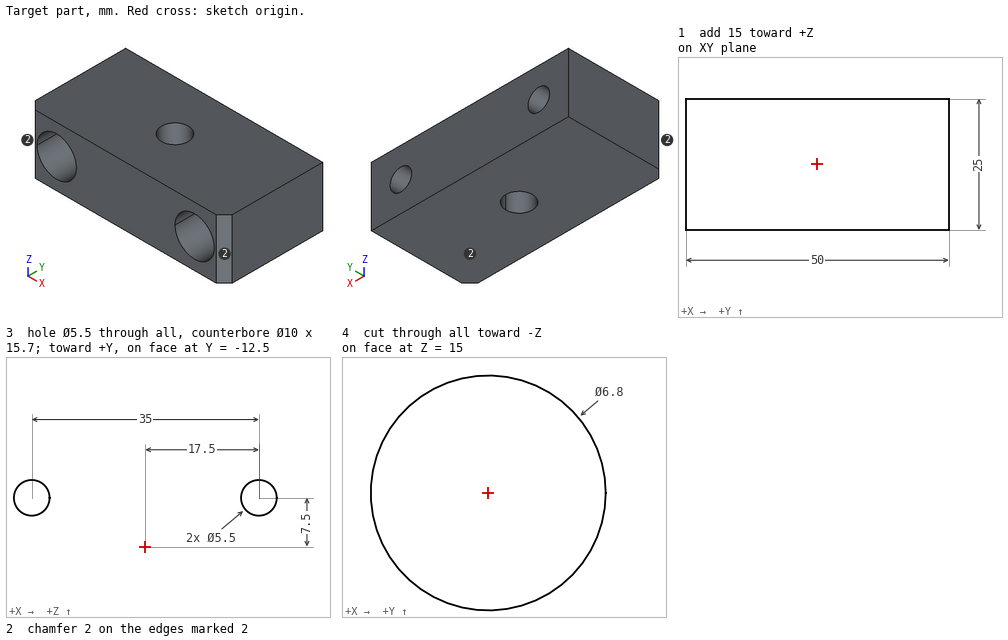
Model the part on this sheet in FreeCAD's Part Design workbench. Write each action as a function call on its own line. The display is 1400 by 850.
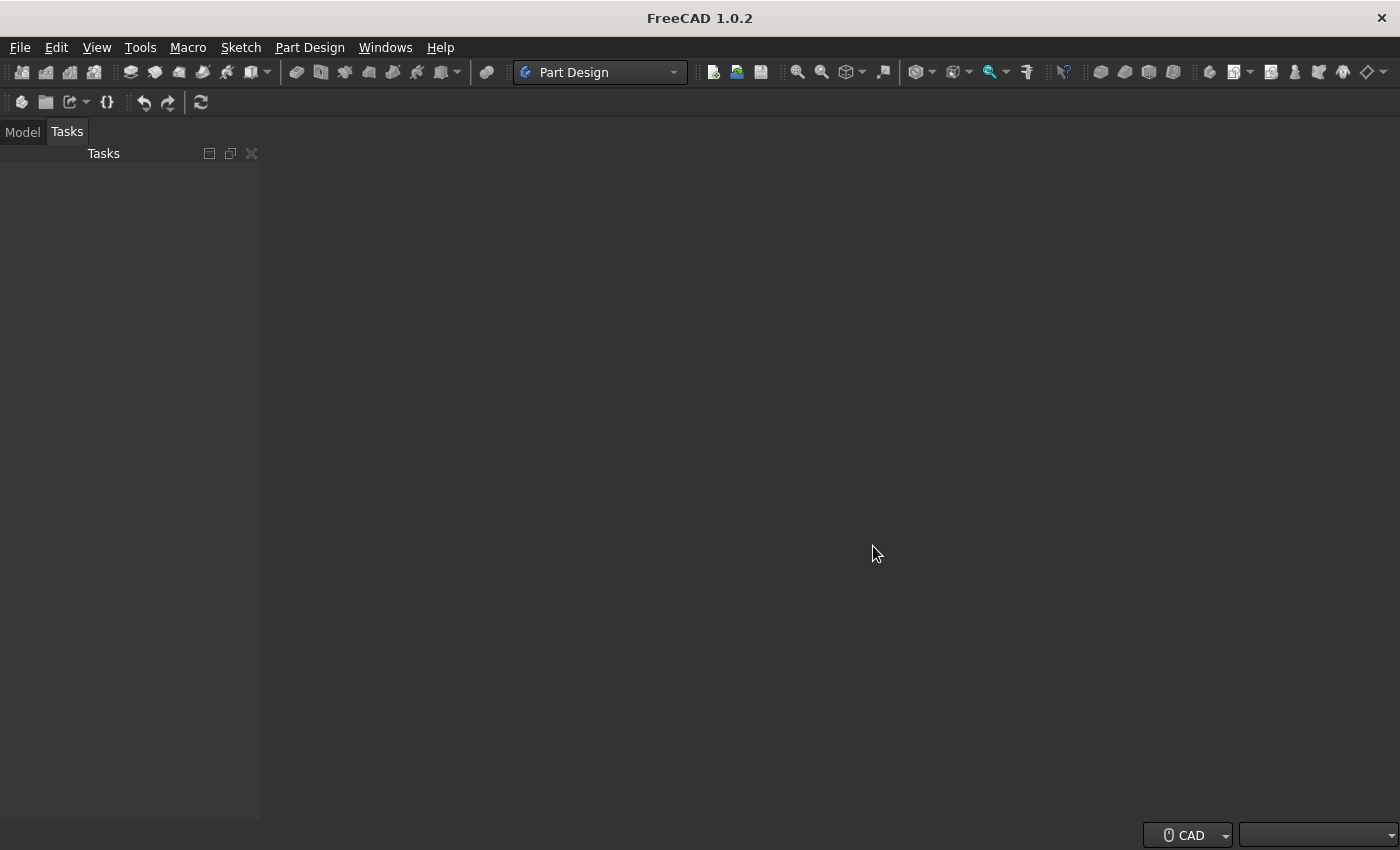
click(714, 72)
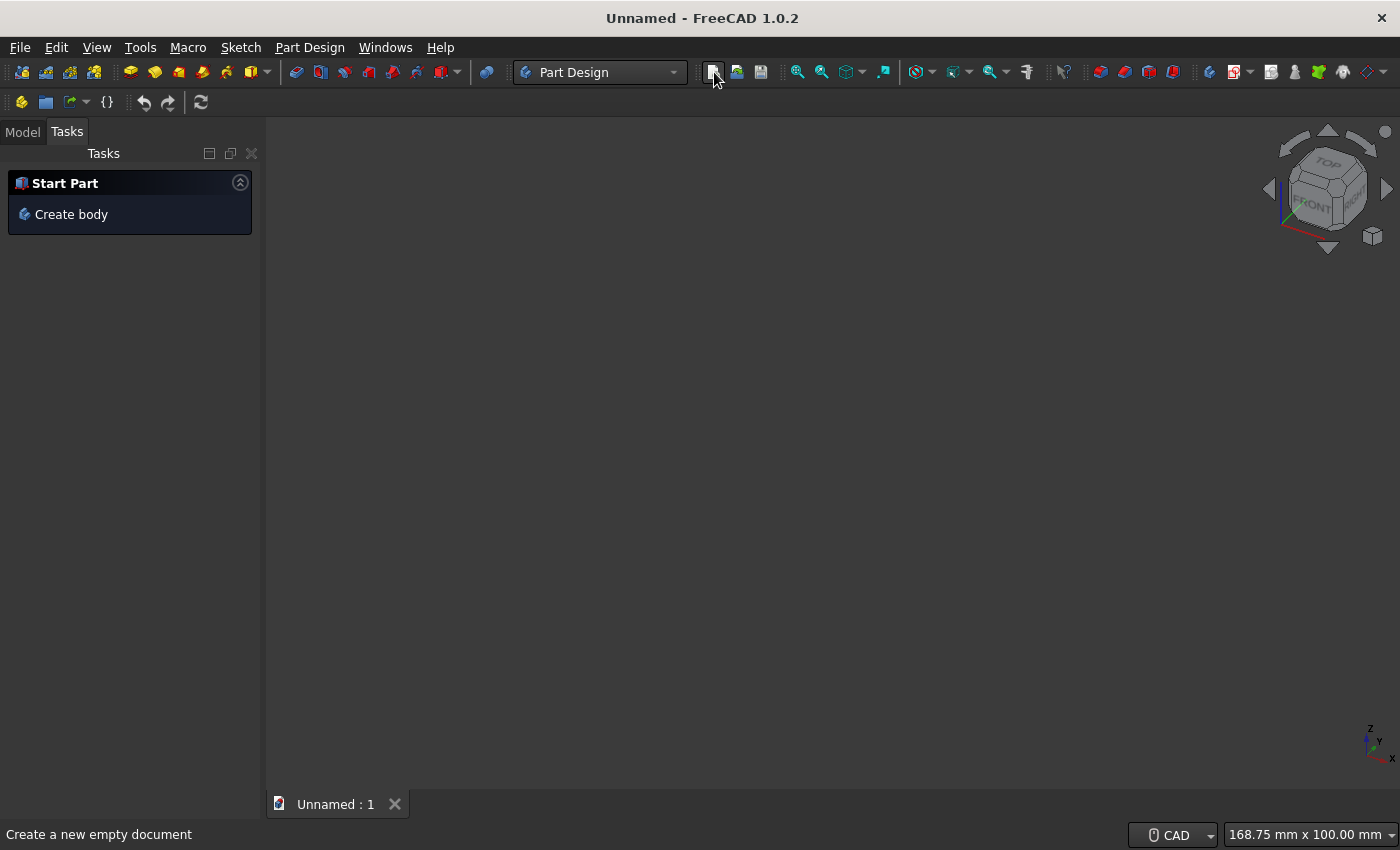
click(1234, 72)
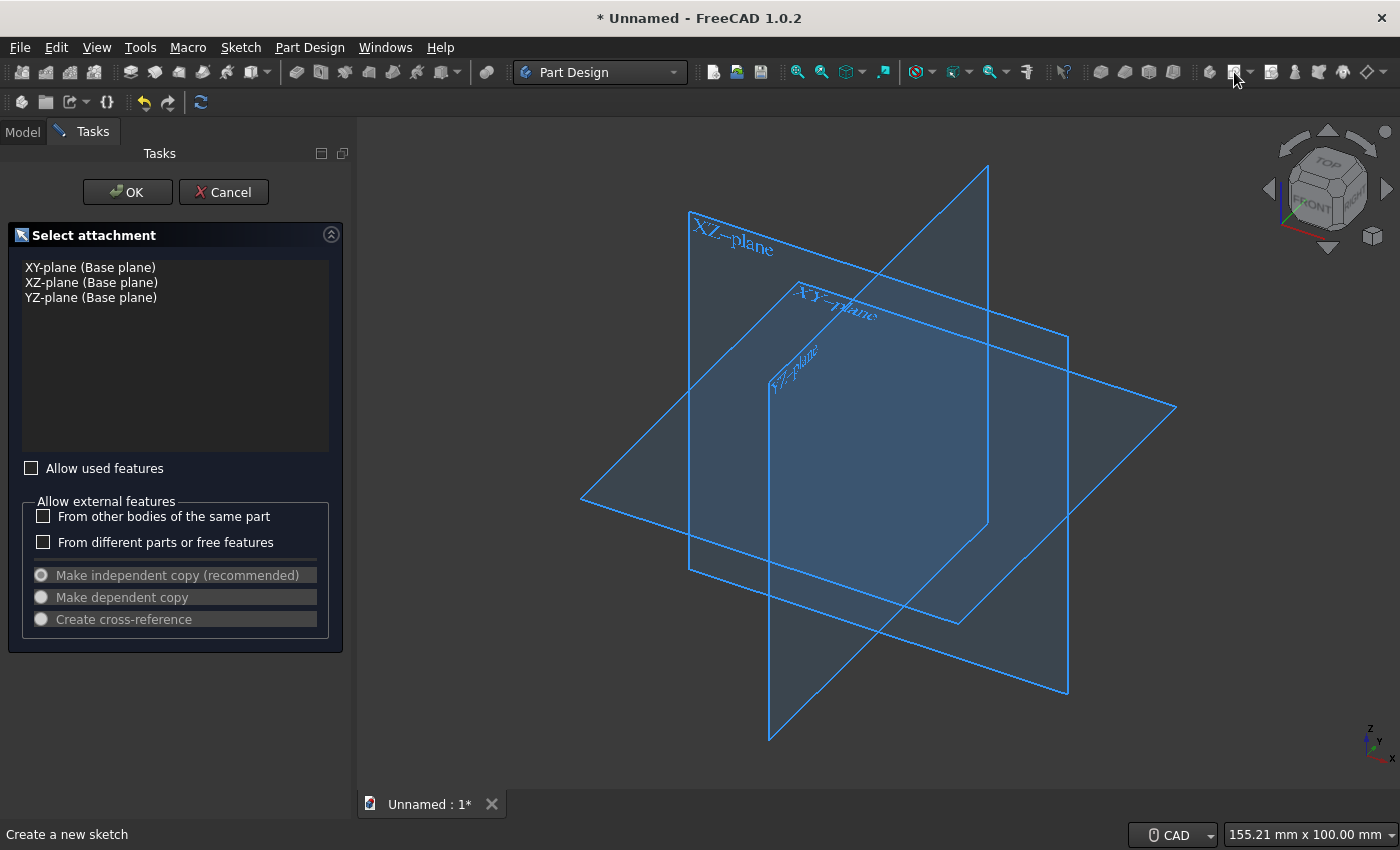
click(82, 268)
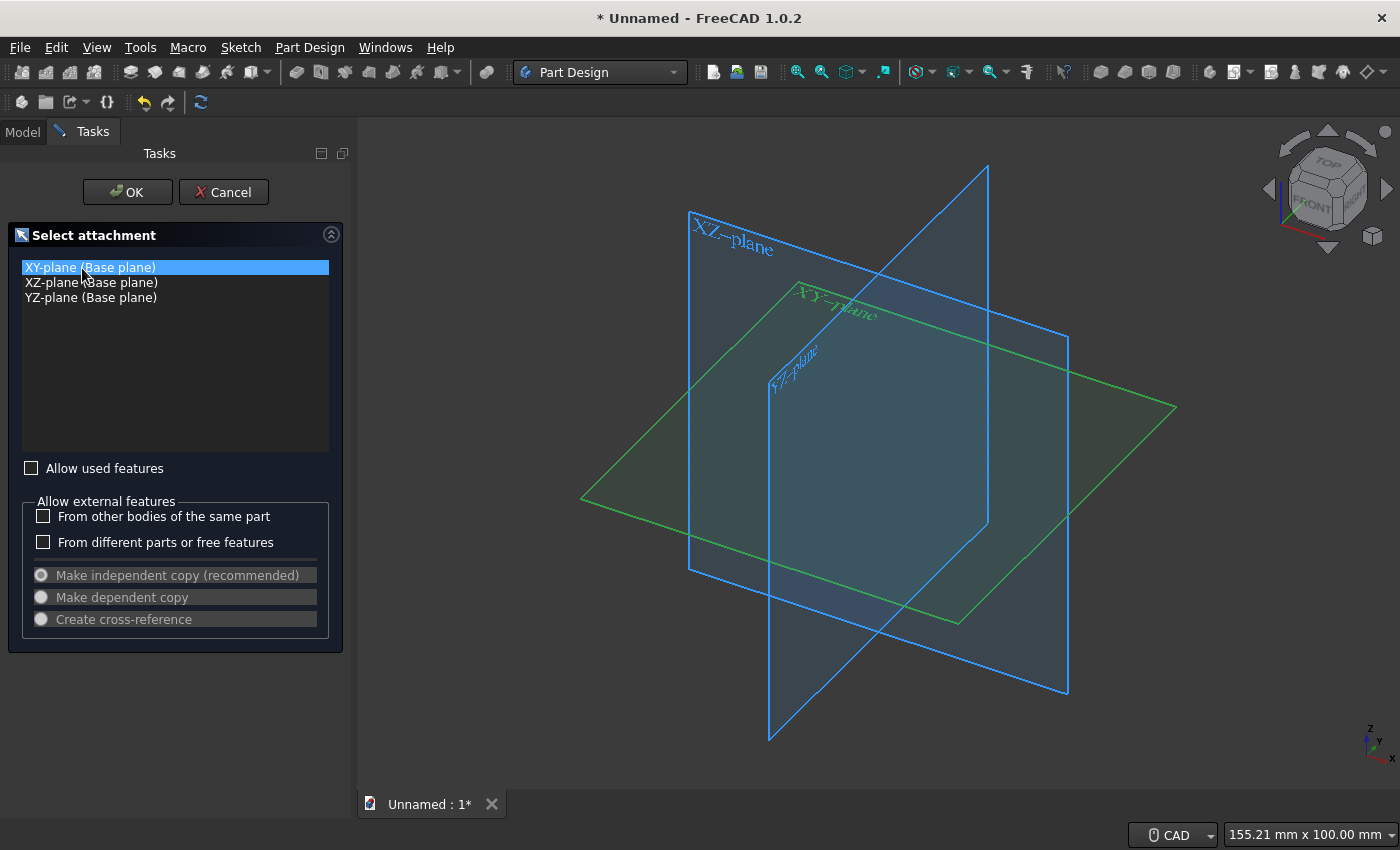
click(128, 192)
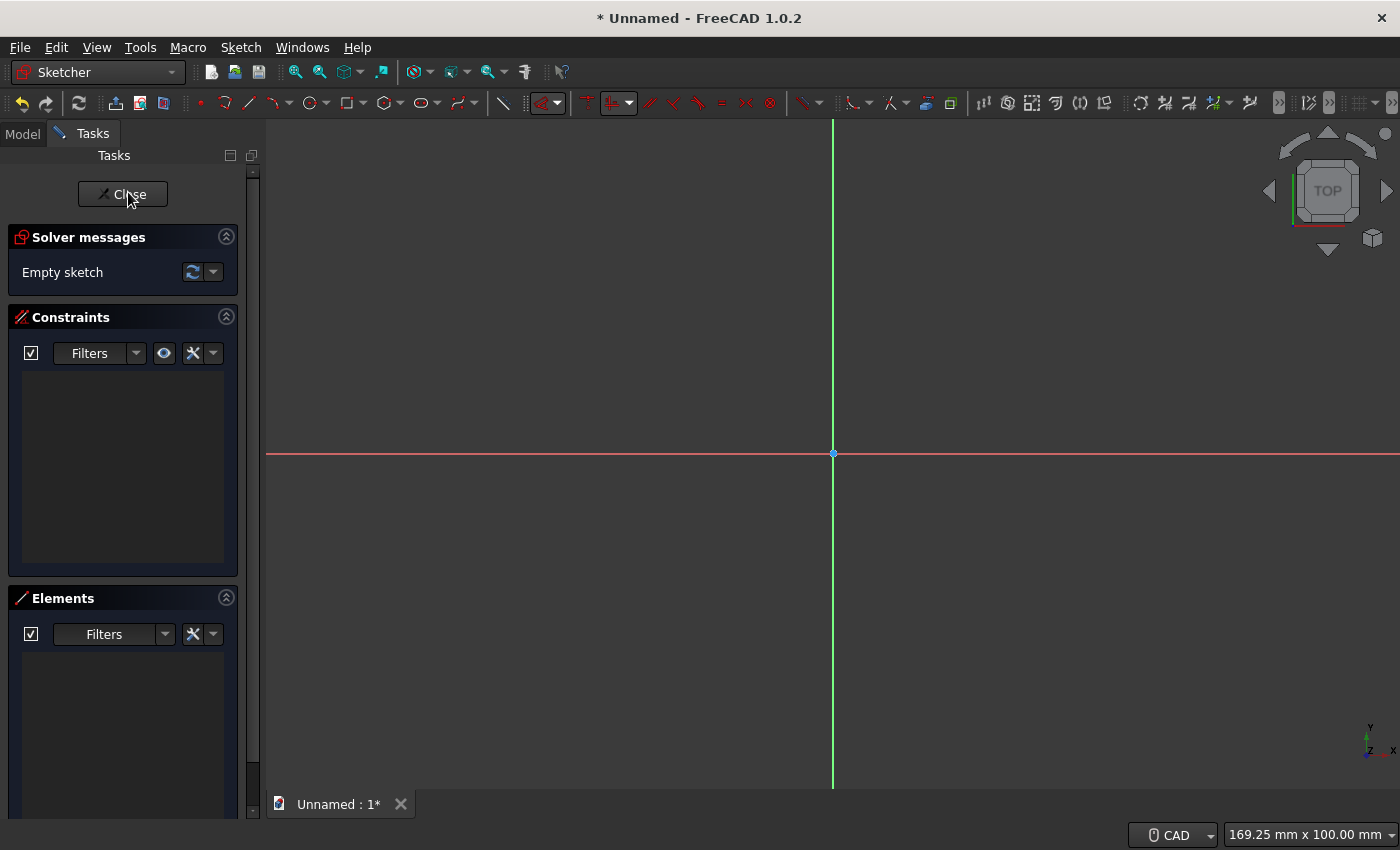
scroll(916, 454, up, 3)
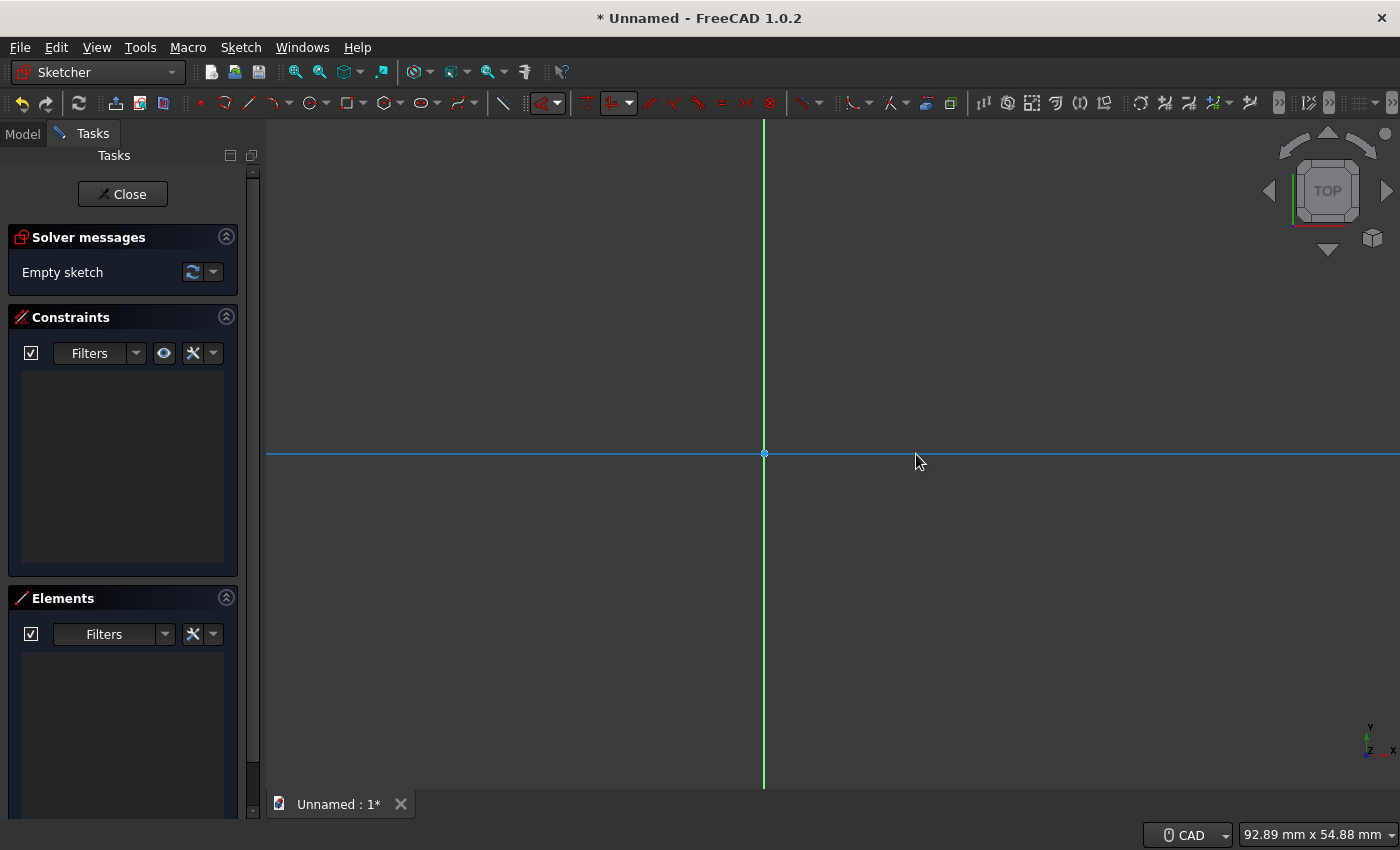
click(366, 104)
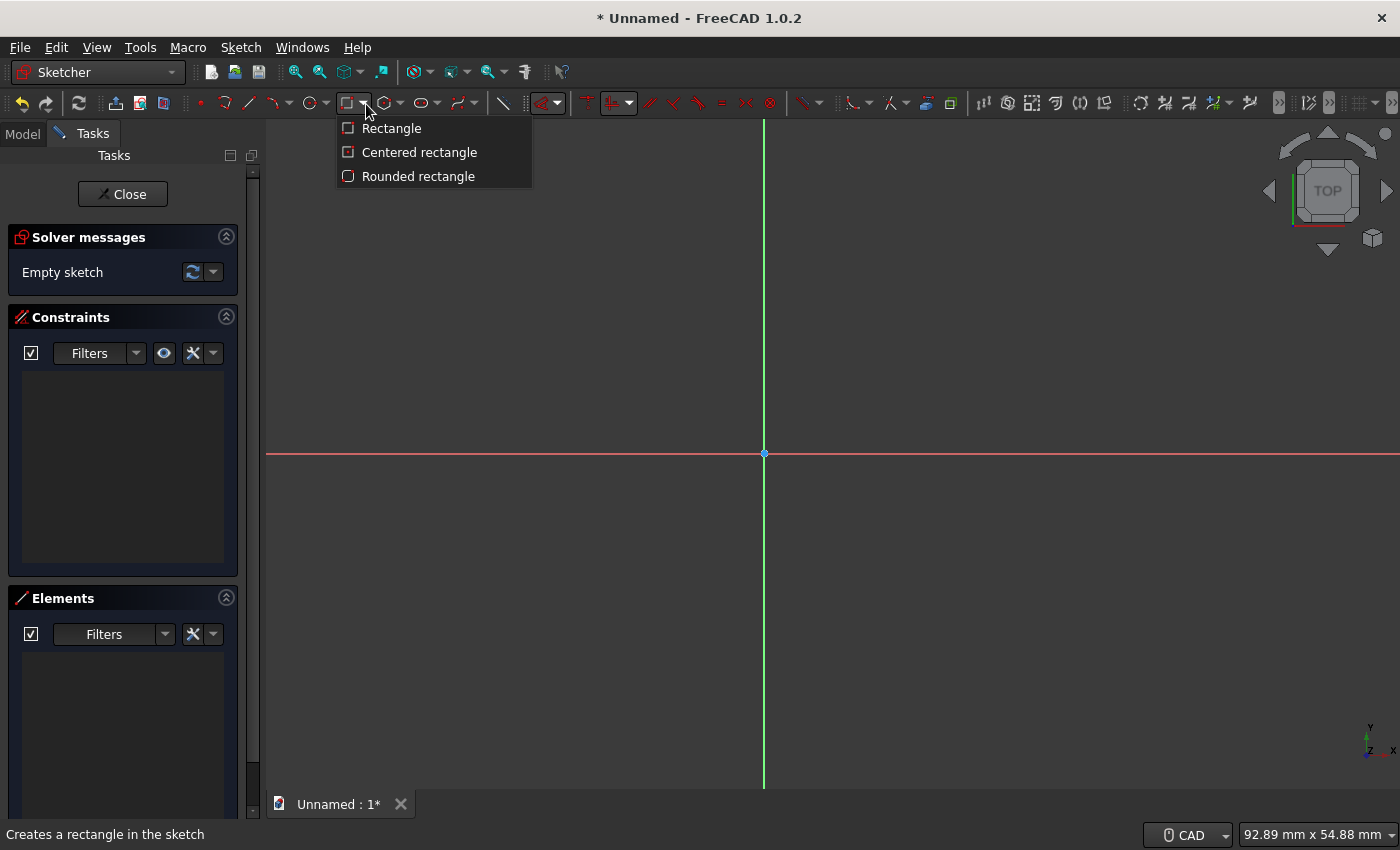
click(434, 152)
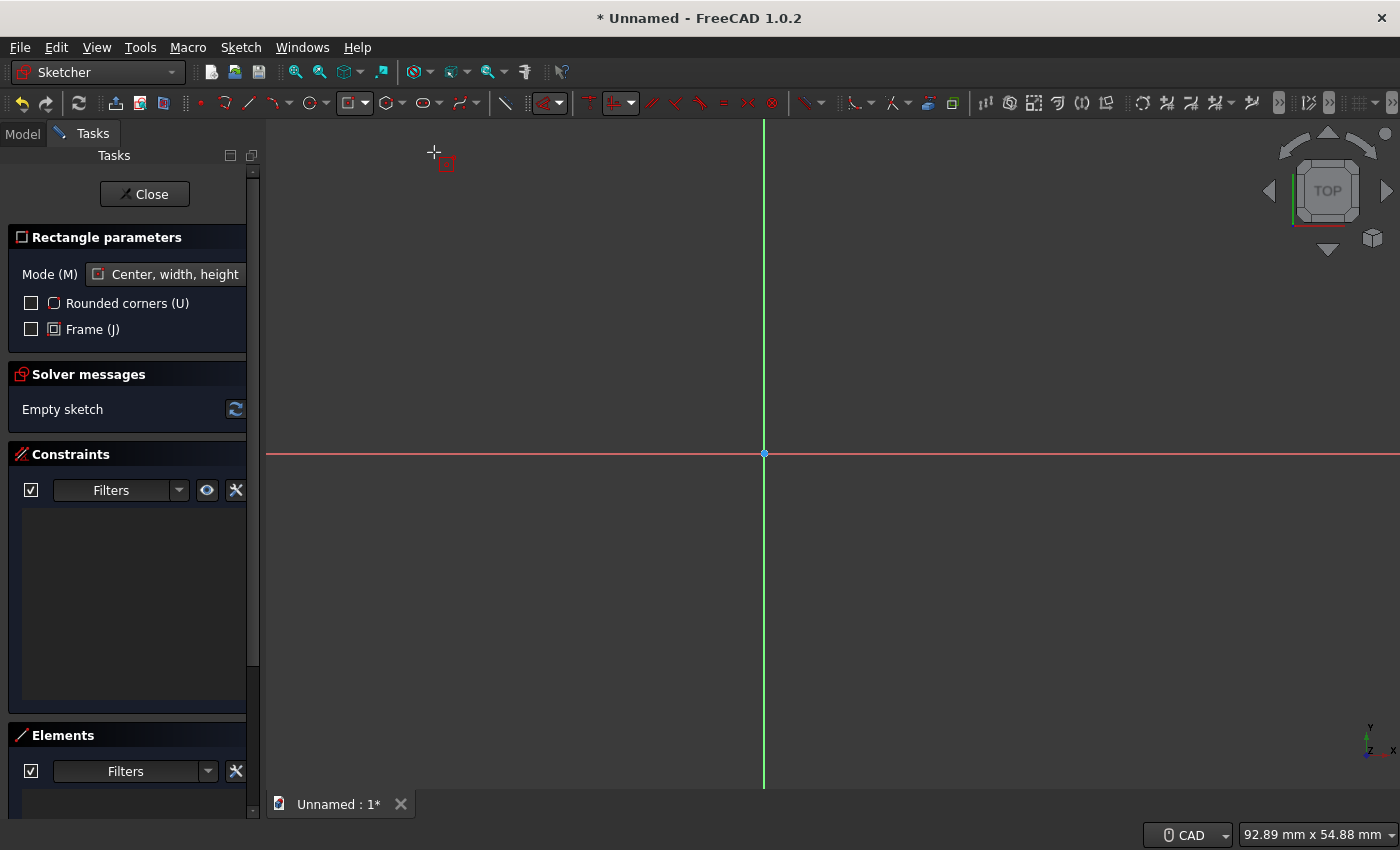
click(764, 454)
move(1069, 301)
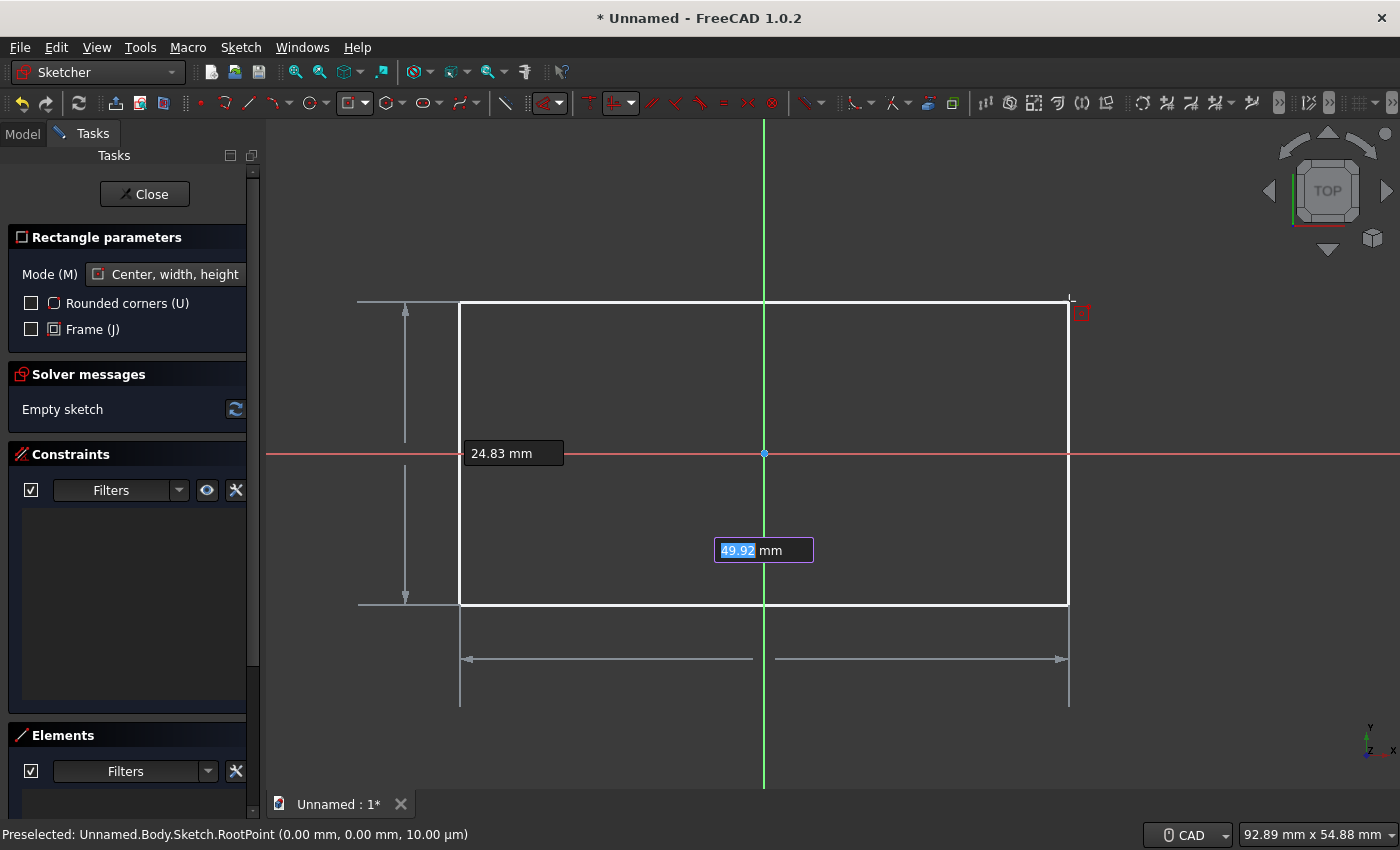
text(50)
key(Tab)
text(25)
key(Return)
key(Escape)